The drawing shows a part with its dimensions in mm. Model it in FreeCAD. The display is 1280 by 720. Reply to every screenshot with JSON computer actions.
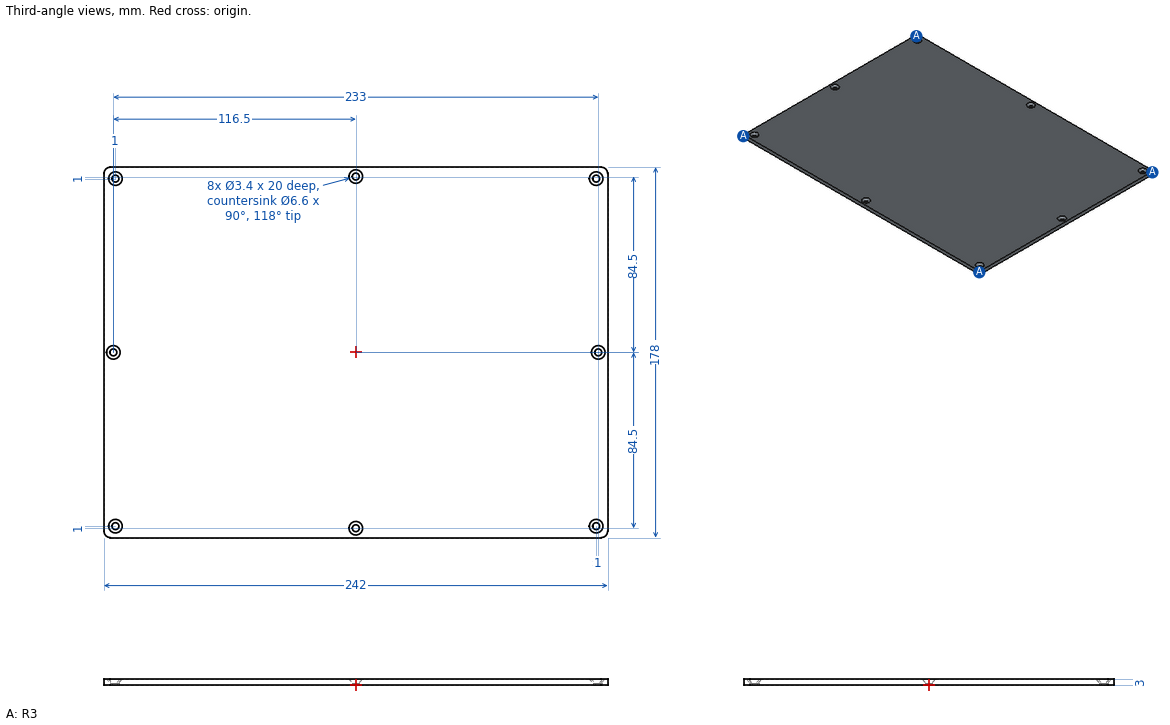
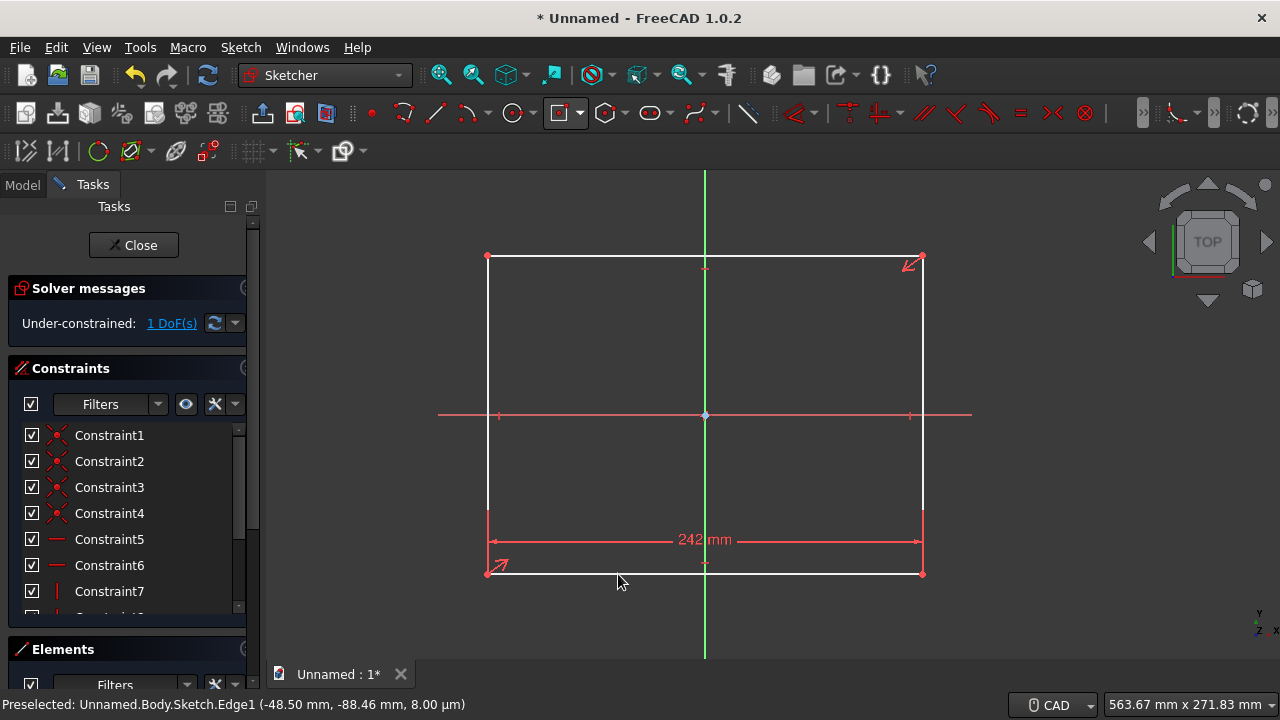
{"action": "left_click", "coordinate": [923, 479]}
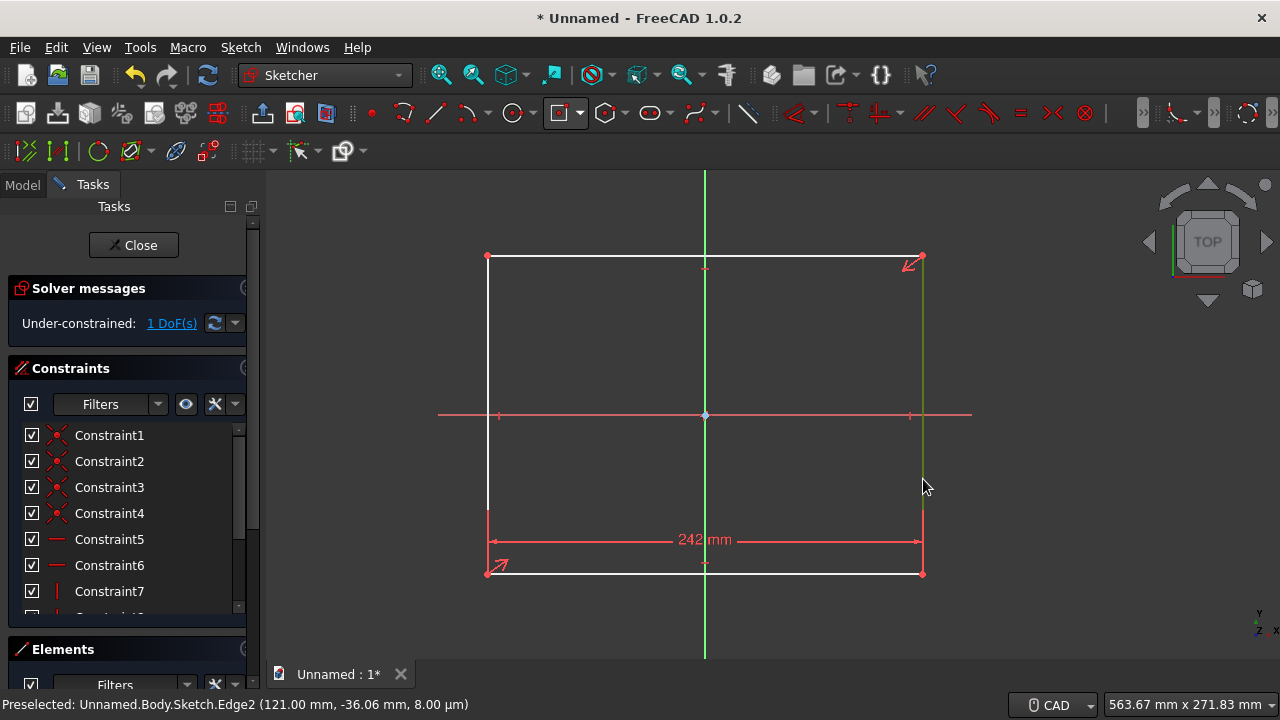
{"action": "key", "text": "i"}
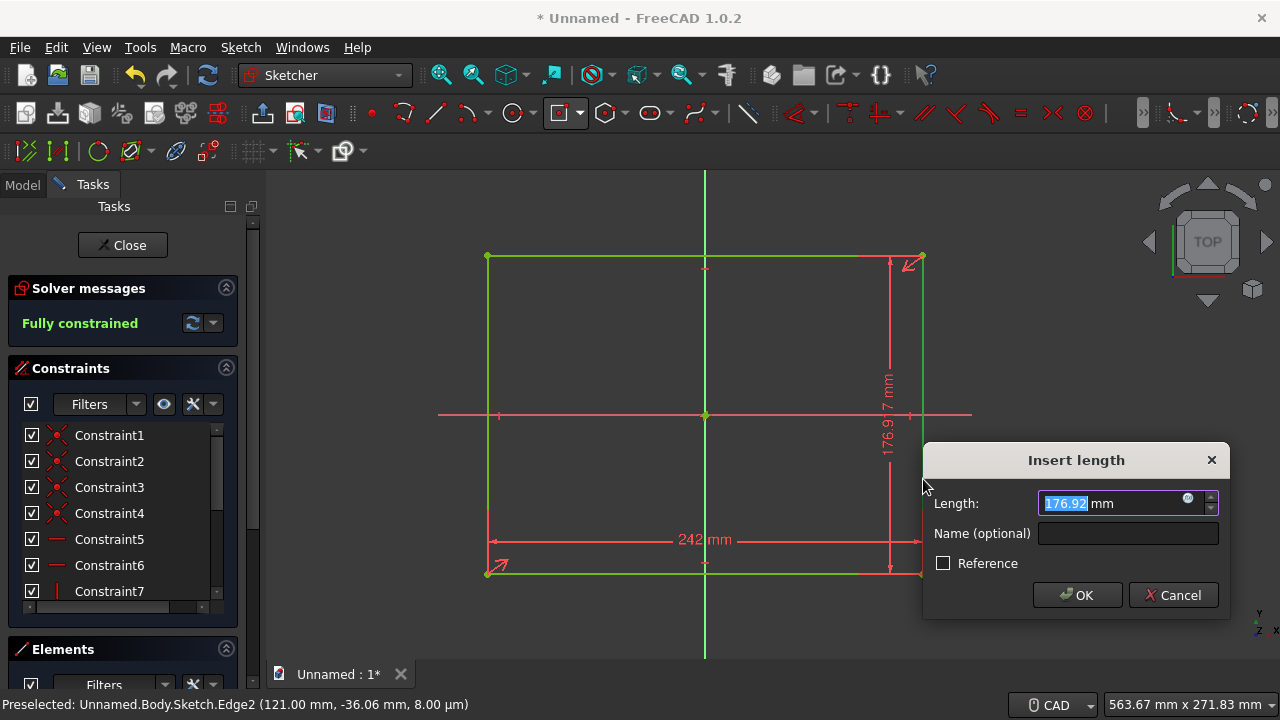
{"action": "type", "text": "178"}
{"action": "key", "text": "Return"}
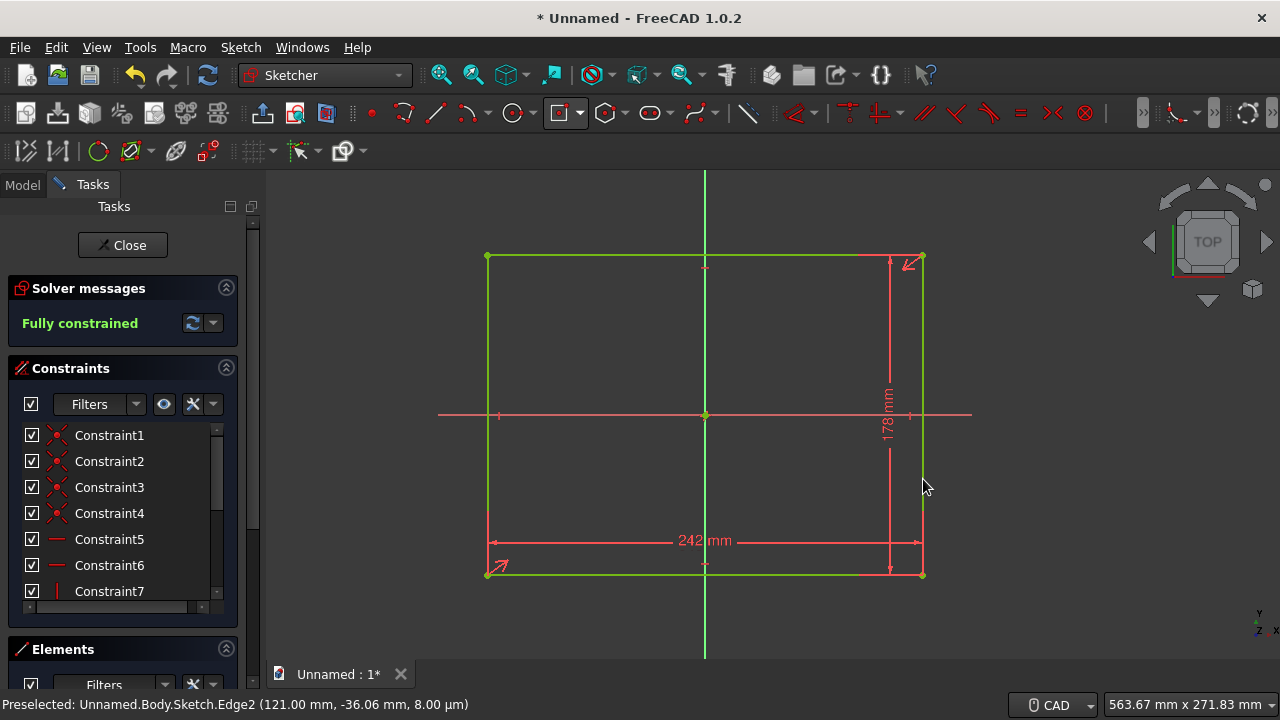
{"action": "left_click", "coordinate": [123, 245]}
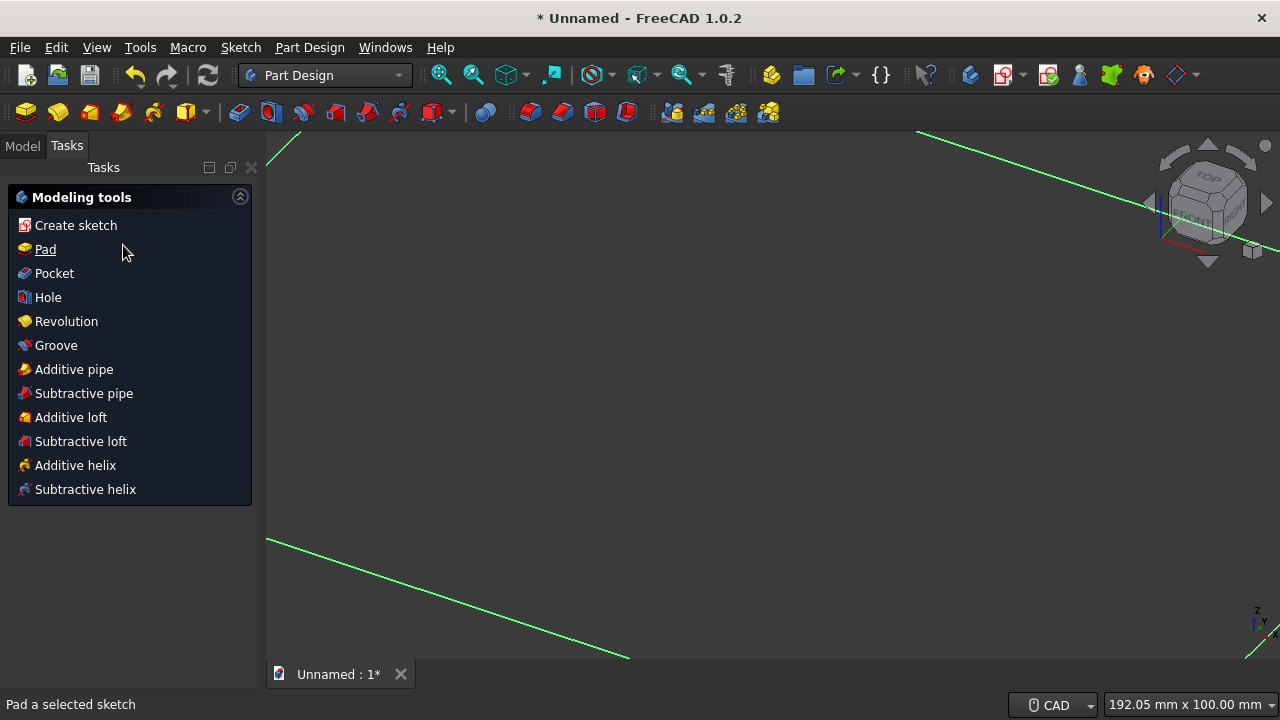
{"action": "left_click", "coordinate": [26, 112]}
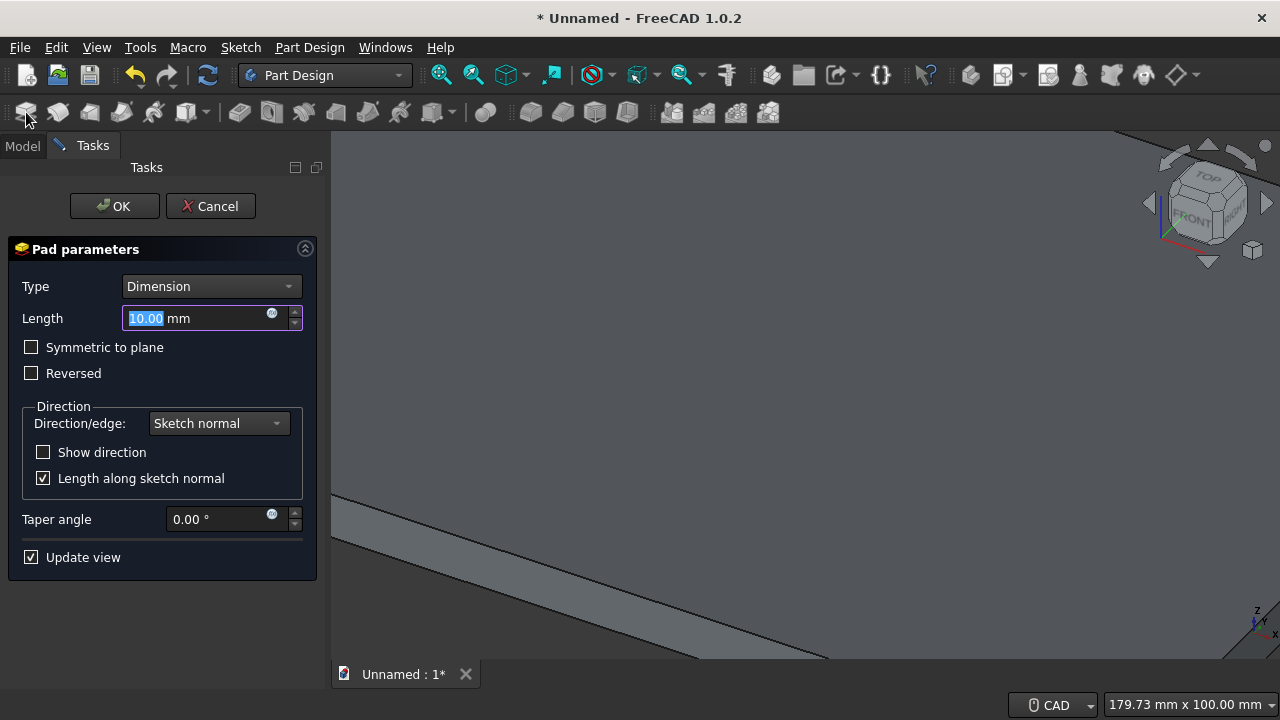
{"action": "type", "text": "3"}
{"action": "key", "text": "Tab"}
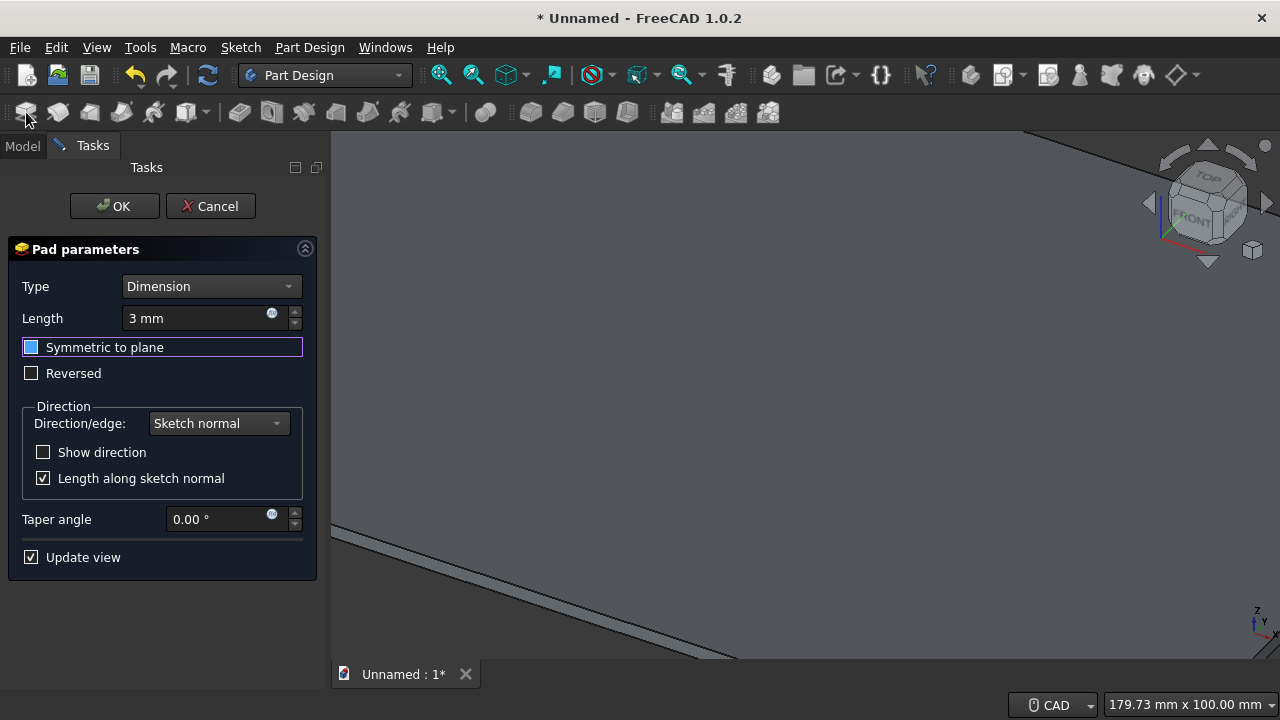
{"action": "left_click", "coordinate": [115, 206]}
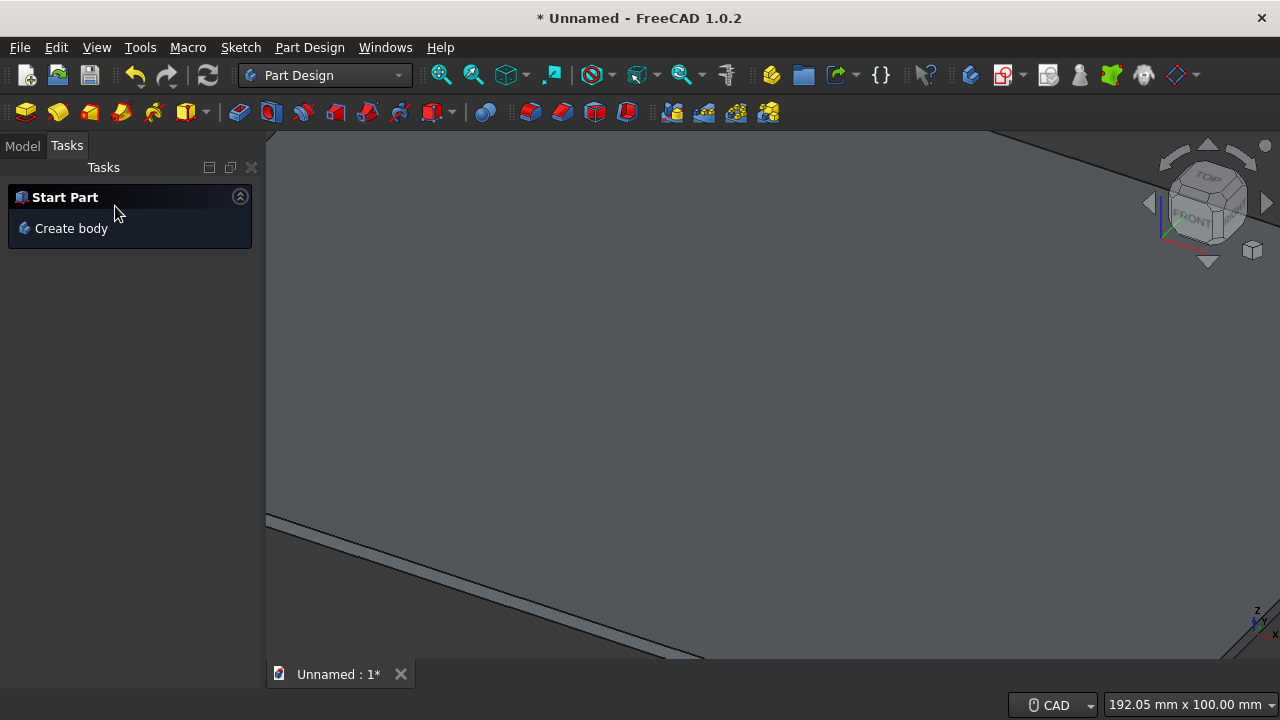
{"action": "left_click", "coordinate": [442, 76]}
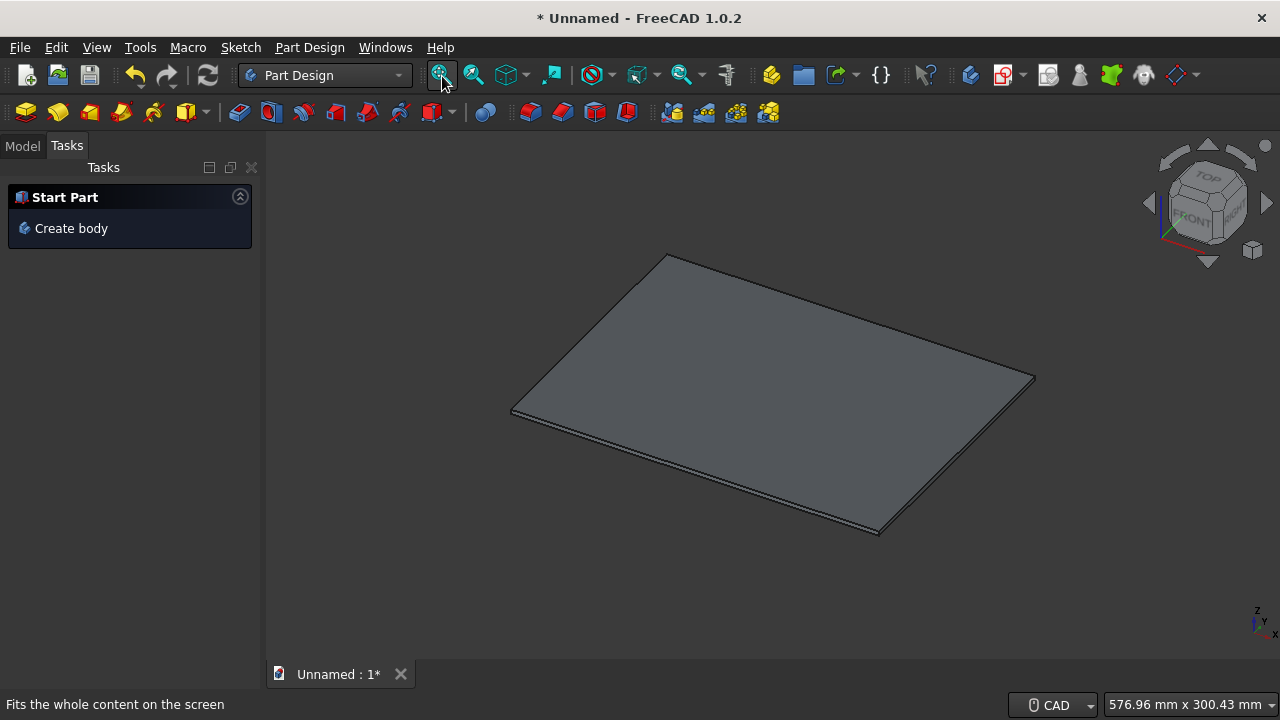
{"action": "scroll", "coordinate": [879, 533], "scroll_direction": "up", "scroll_amount": 11}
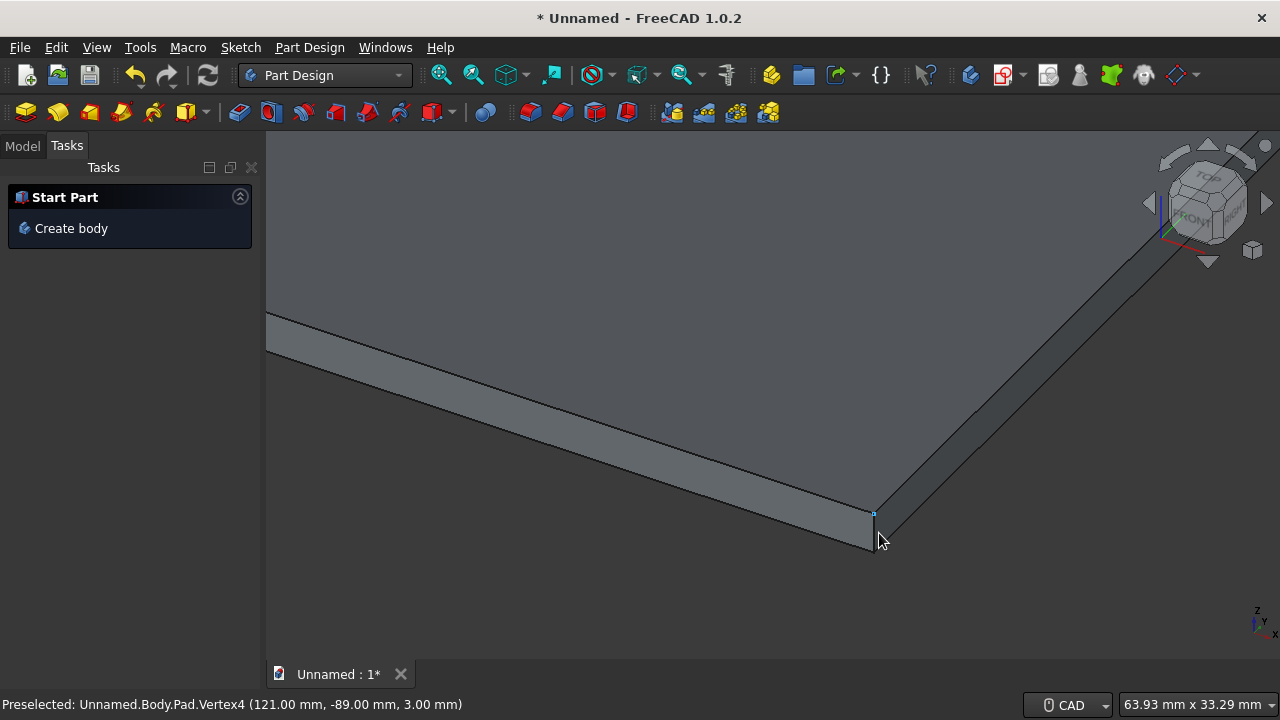
{"action": "left_click", "coordinate": [874, 532]}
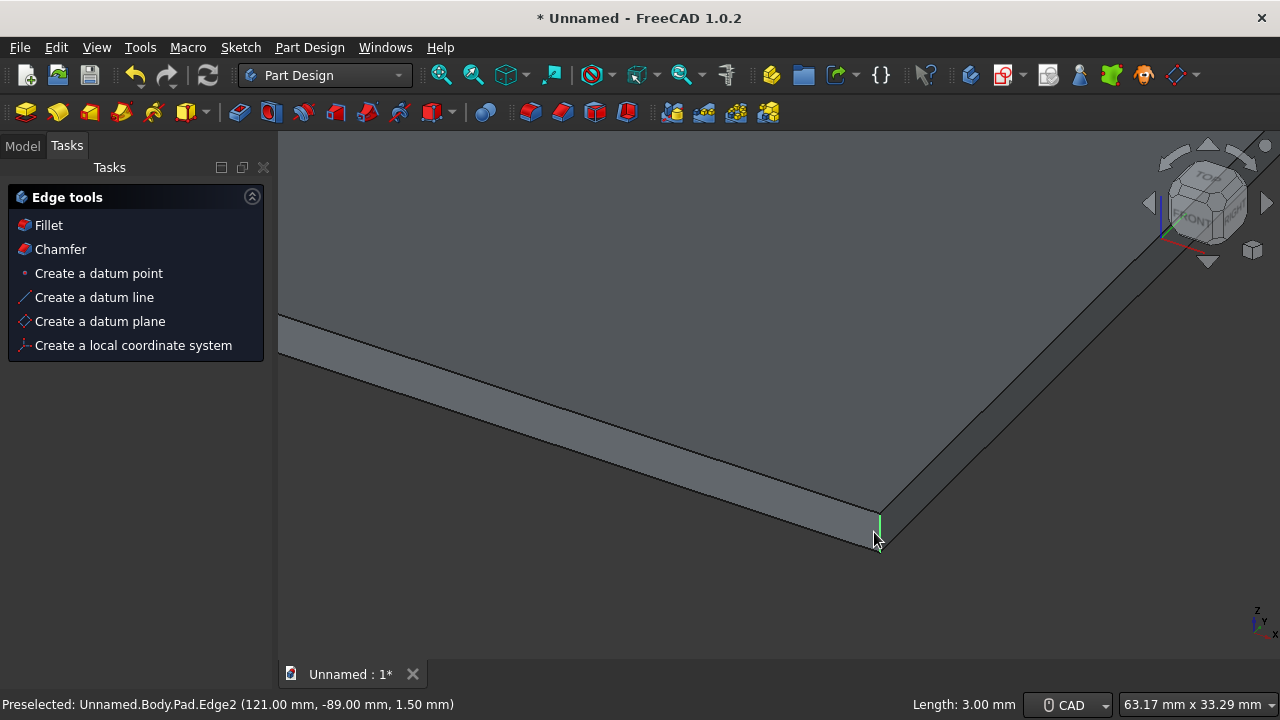
{"action": "left_click", "coordinate": [442, 76]}